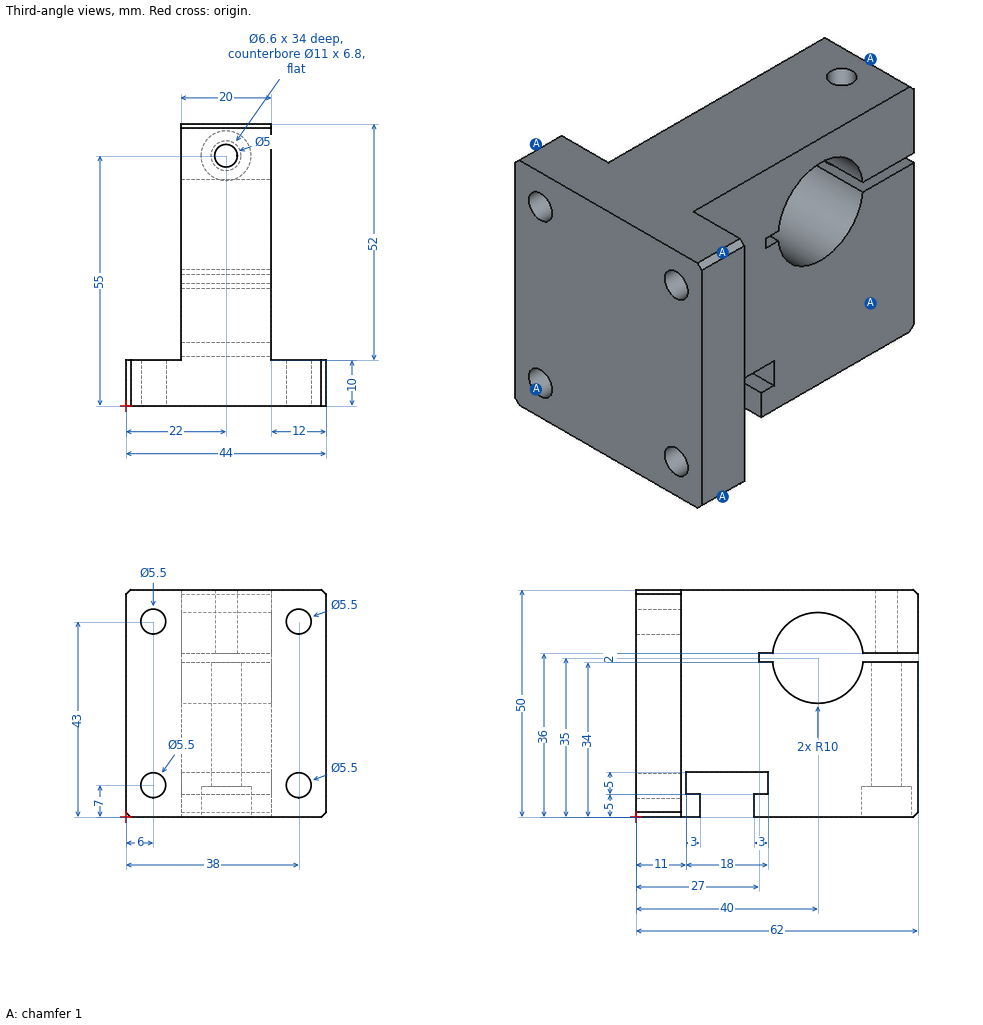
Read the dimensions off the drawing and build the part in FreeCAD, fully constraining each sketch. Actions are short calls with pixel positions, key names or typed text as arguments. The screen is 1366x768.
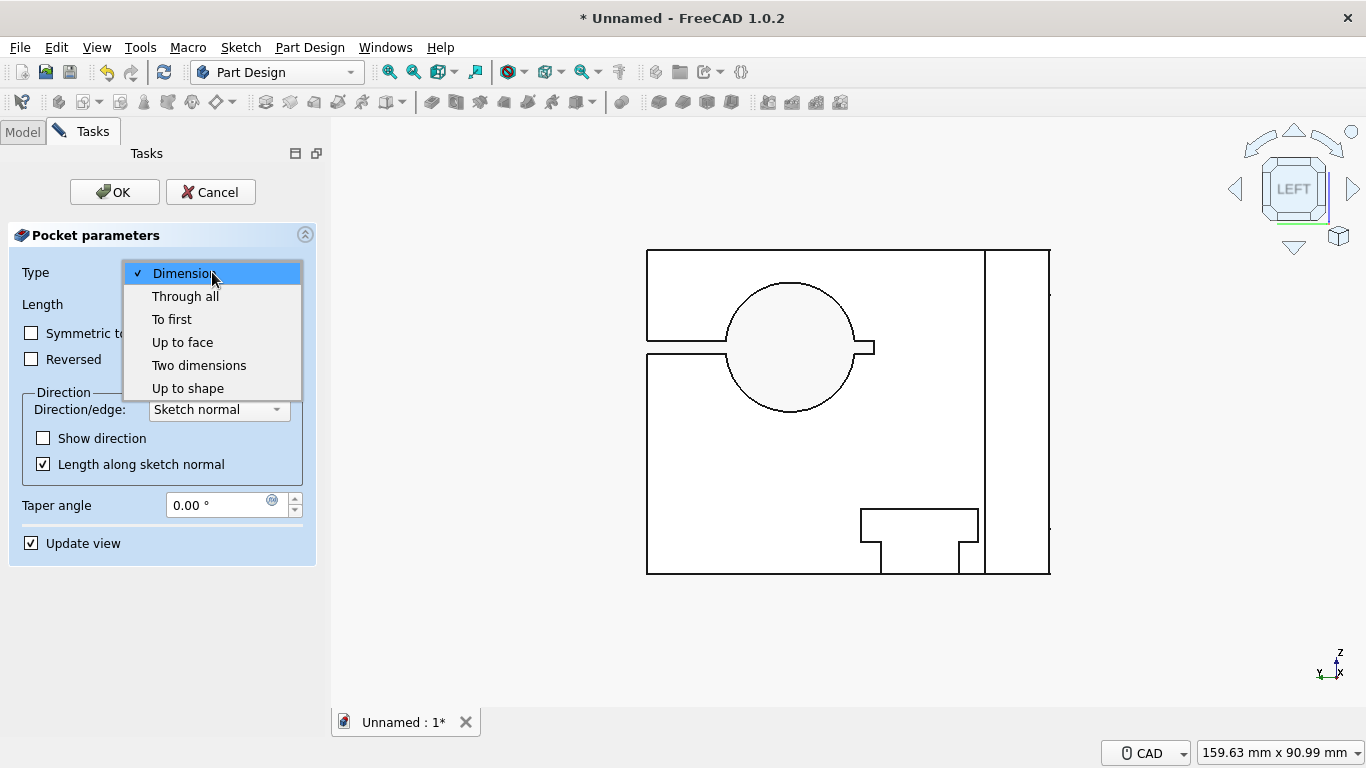
click(212, 320)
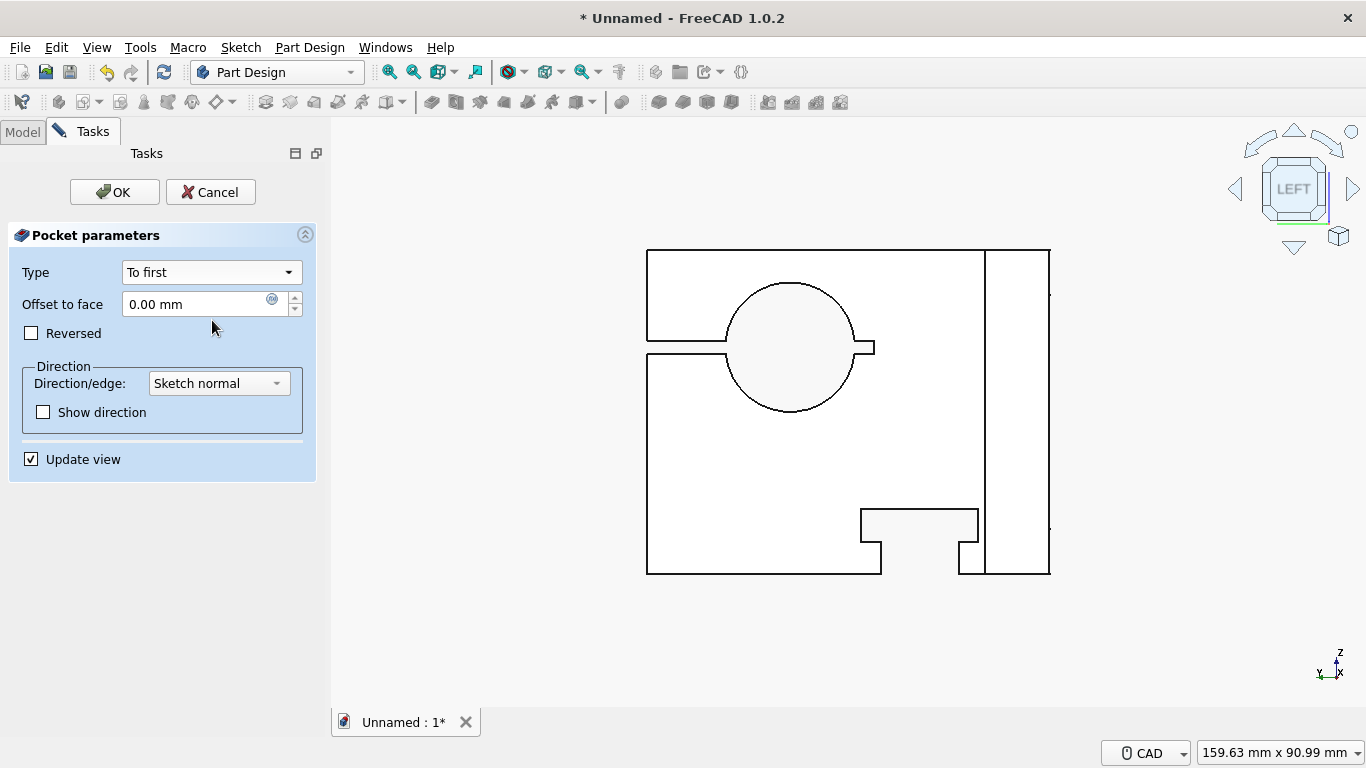
click(115, 192)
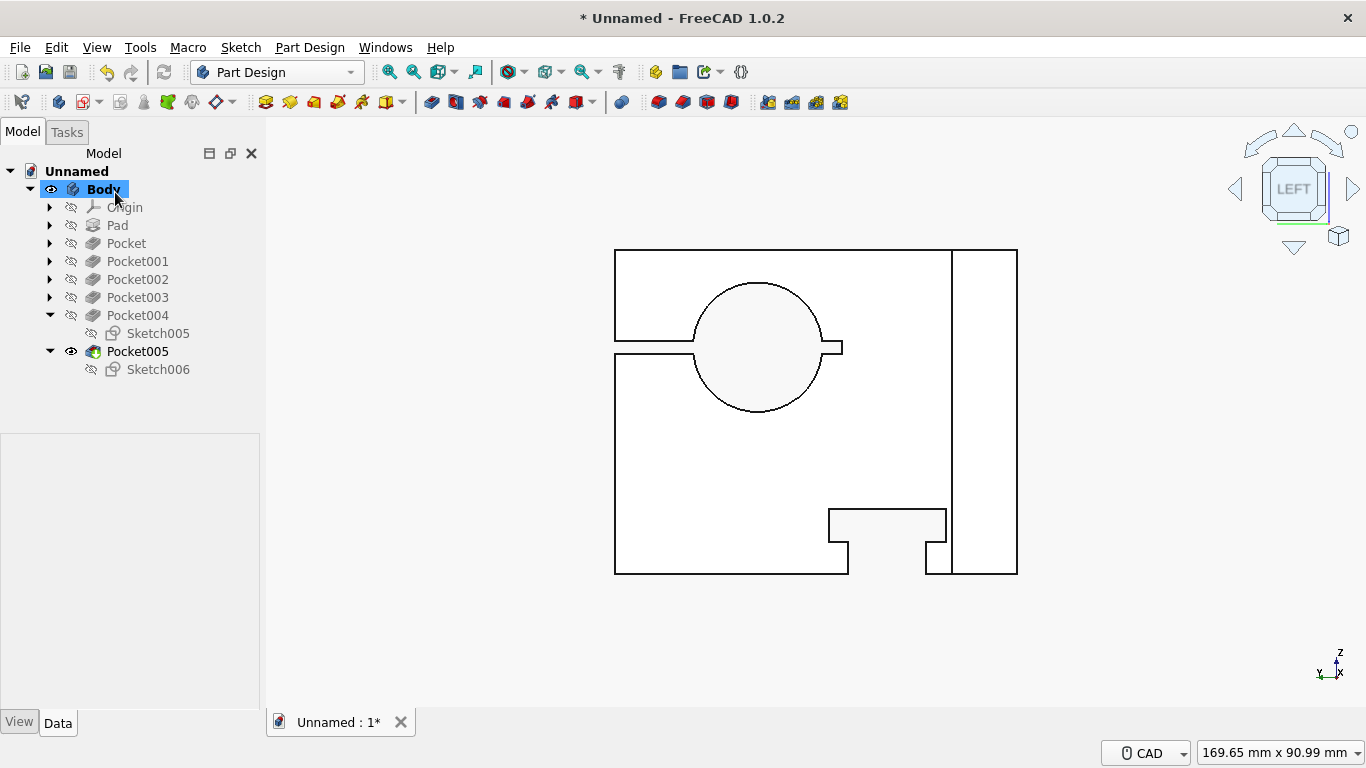
click(84, 102)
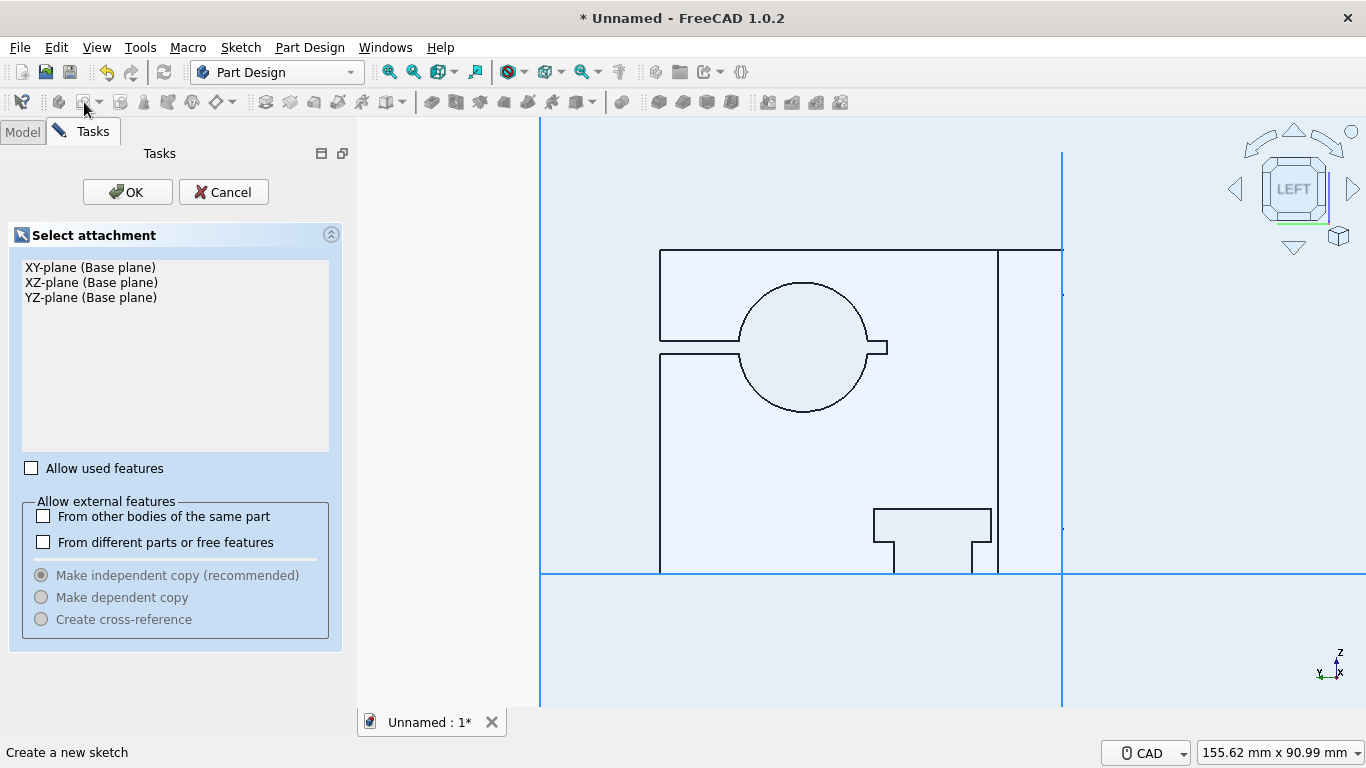
click(82, 268)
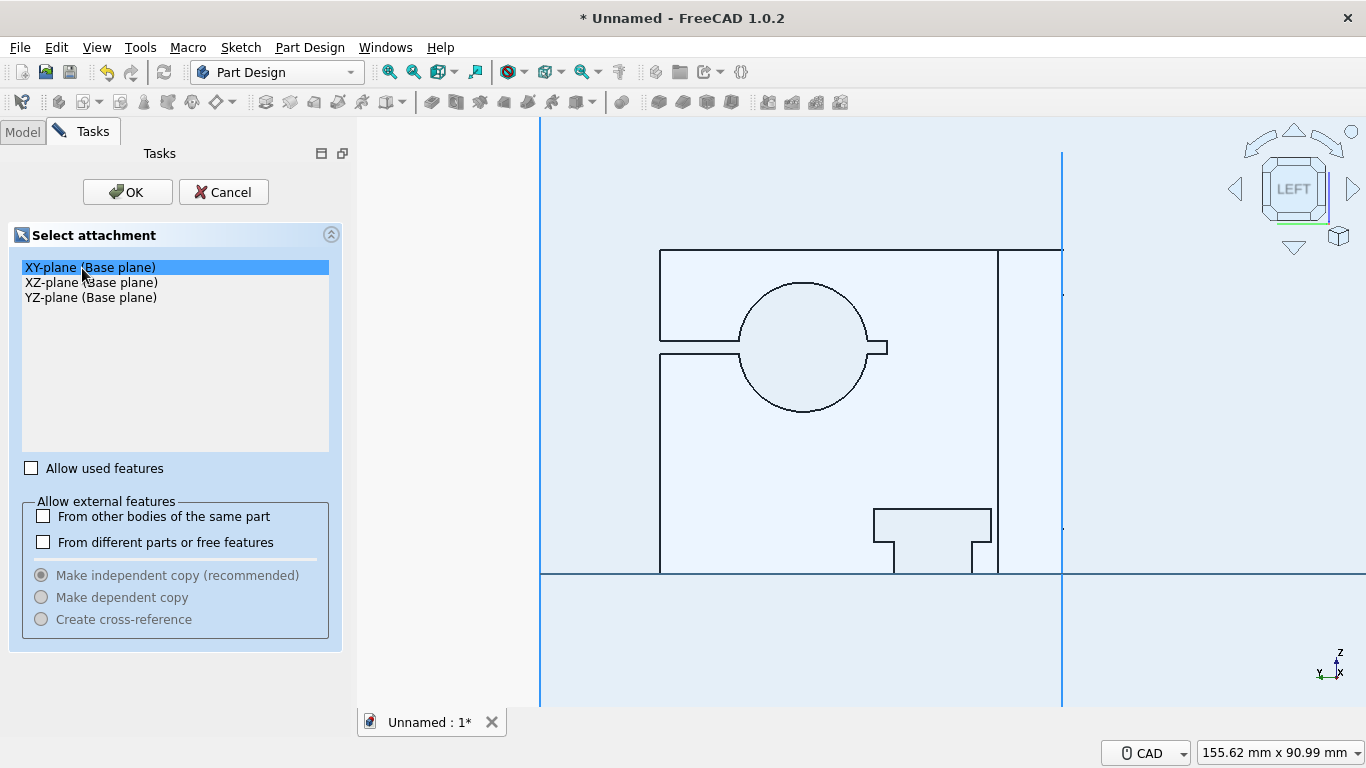
click(128, 192)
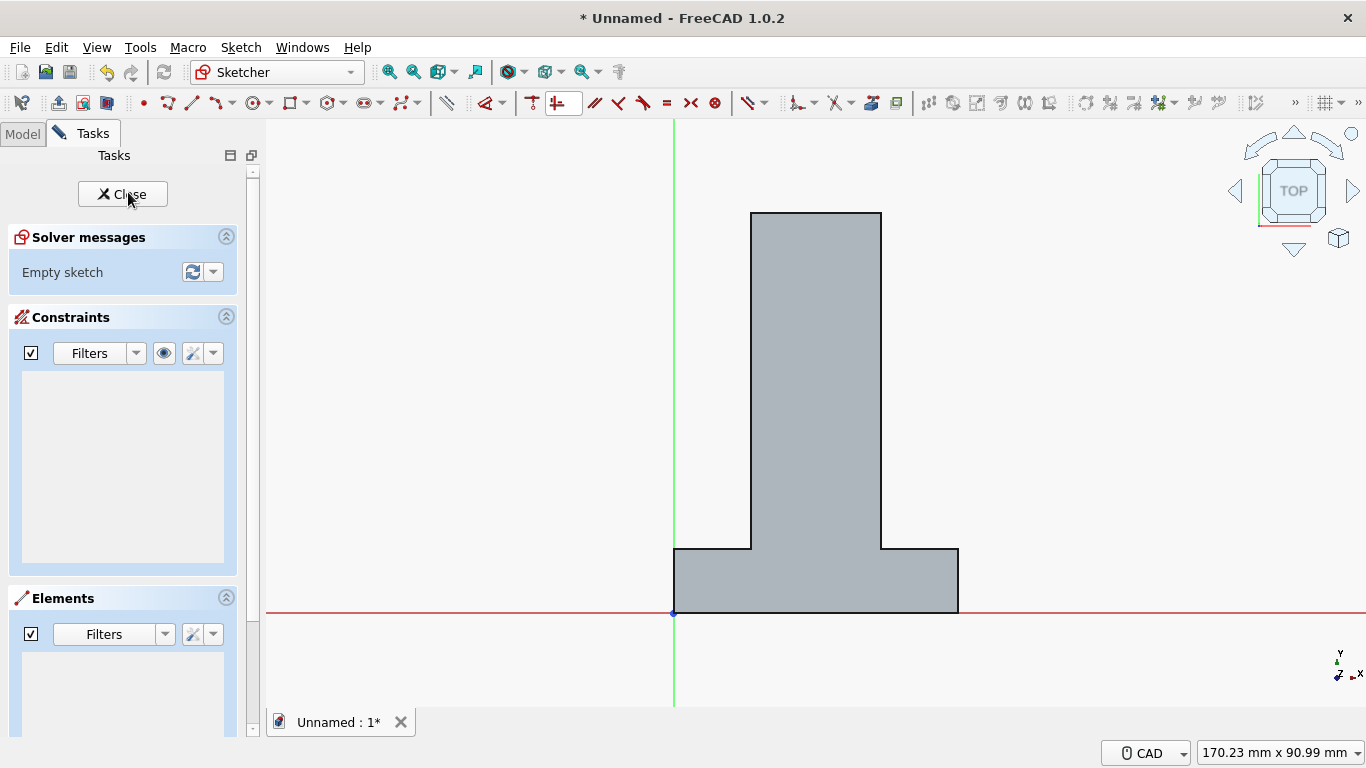
click(108, 104)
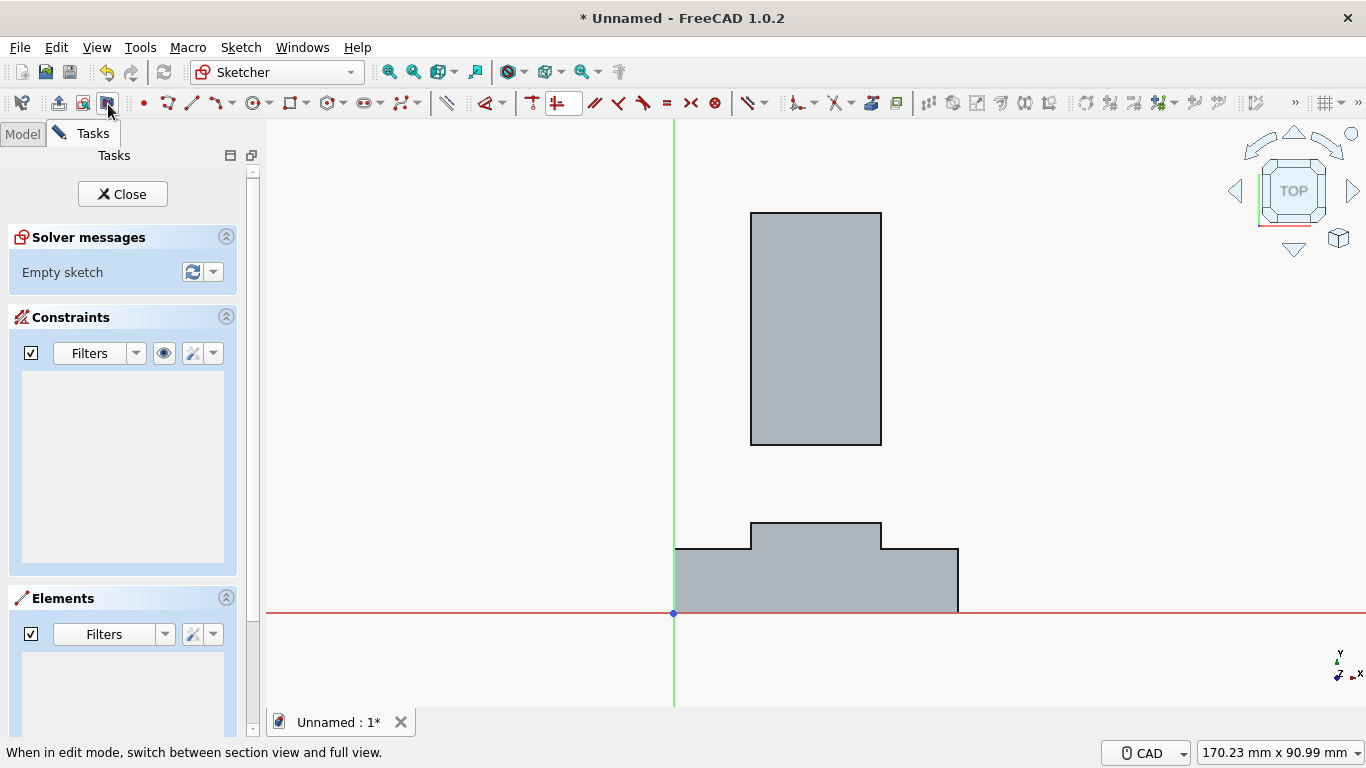
scroll(825, 239, up, 11)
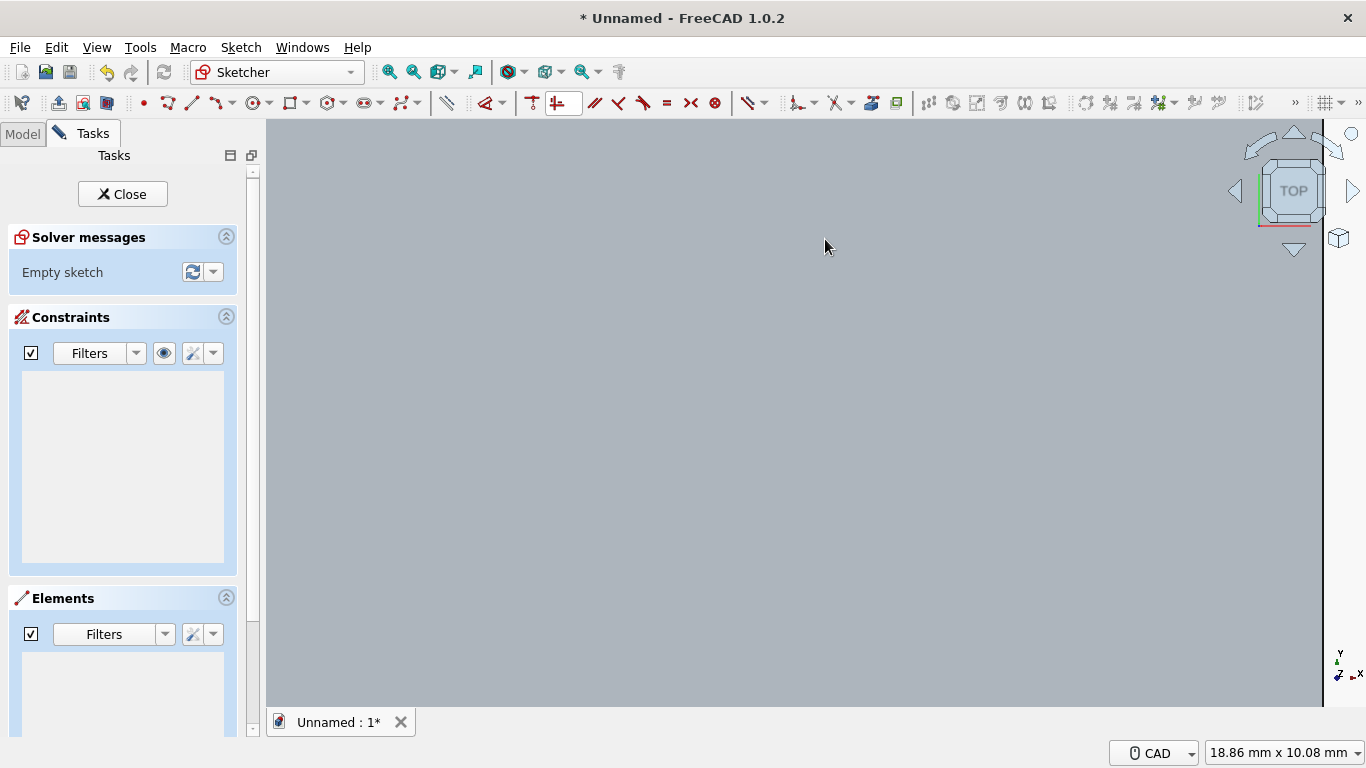
click(254, 104)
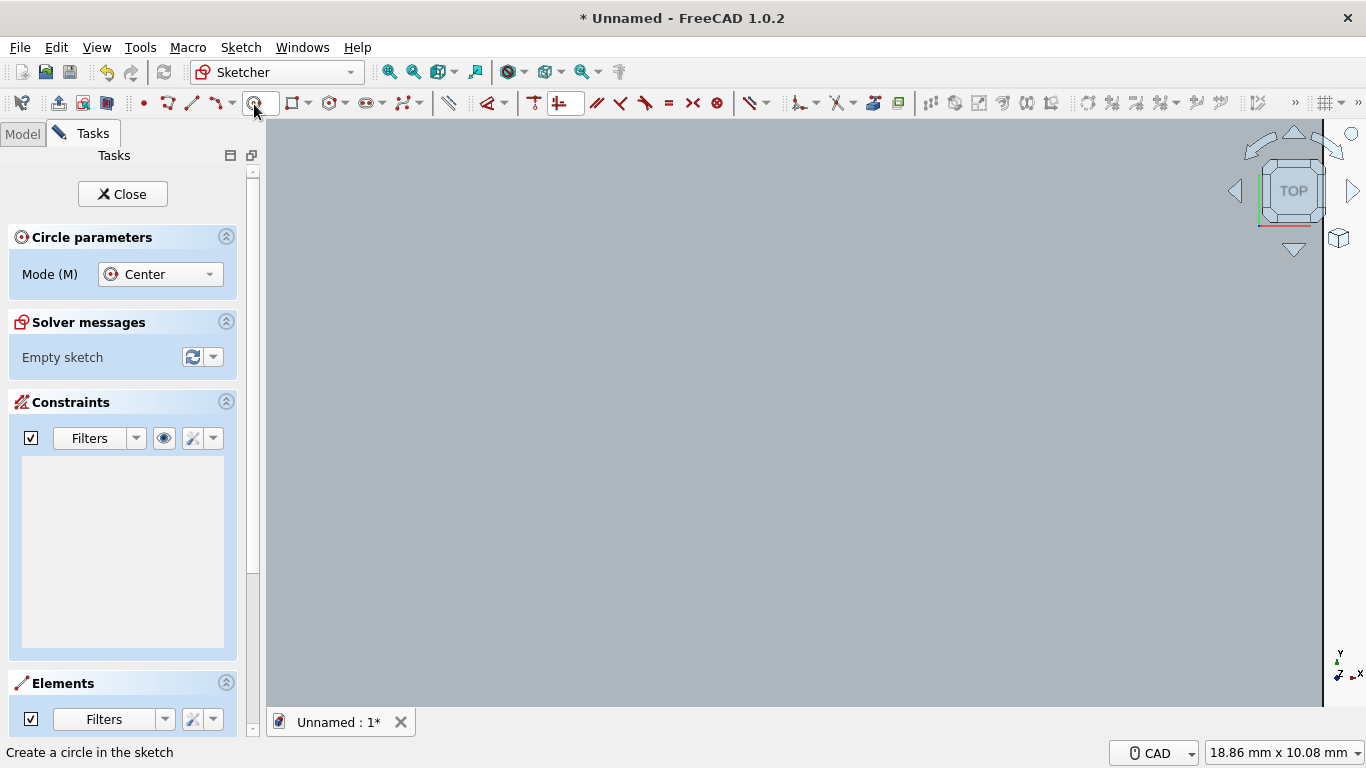
click(740, 408)
move(876, 272)